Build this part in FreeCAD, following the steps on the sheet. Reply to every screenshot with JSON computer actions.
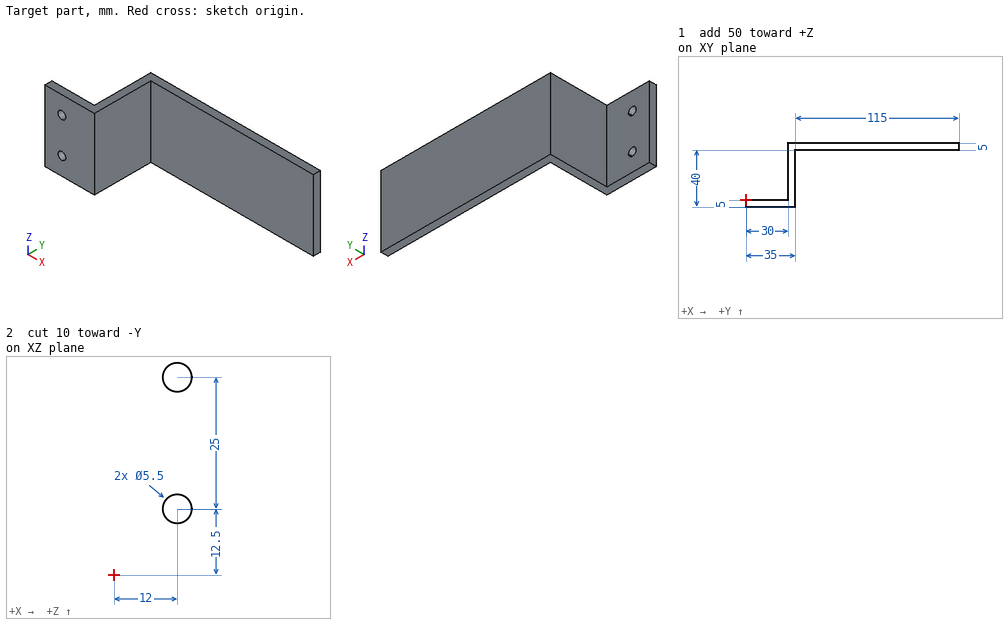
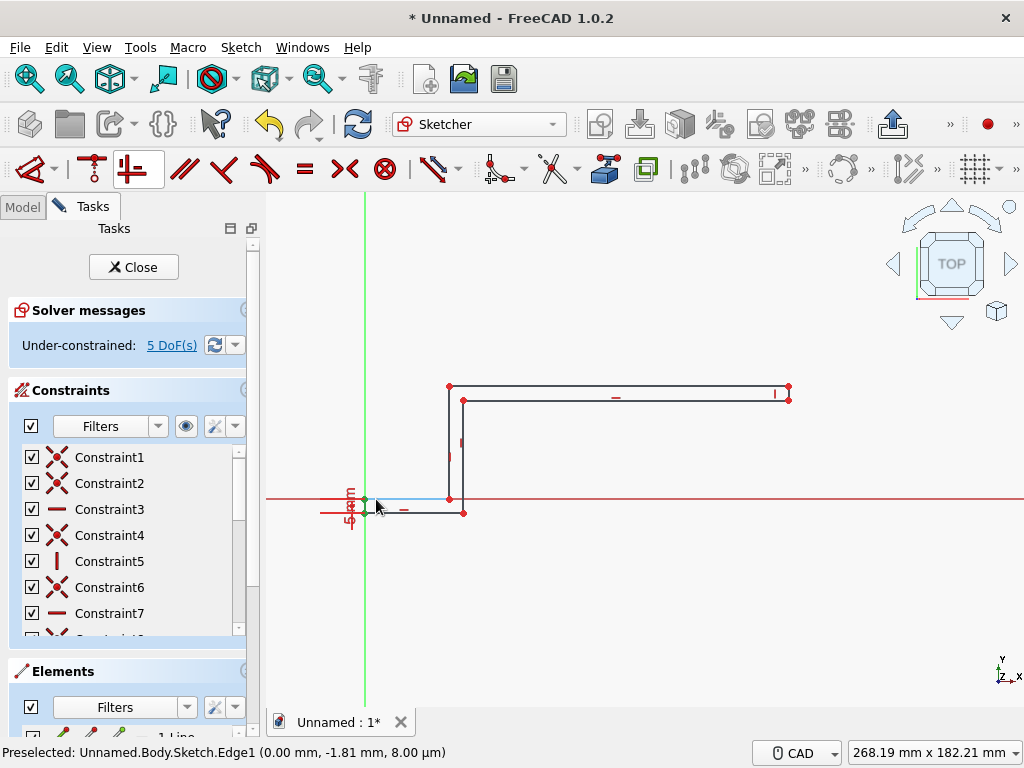
{"action": "scroll", "coordinate": [789, 396], "scroll_direction": "up", "scroll_amount": 6}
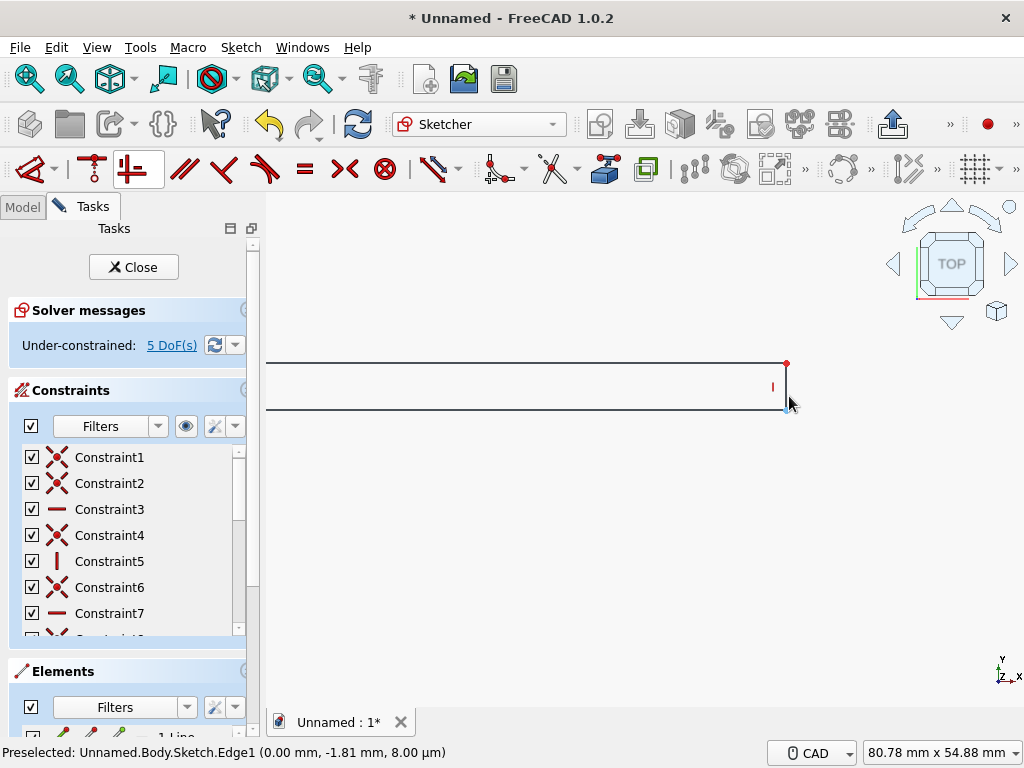
{"action": "left_click", "coordinate": [786, 396]}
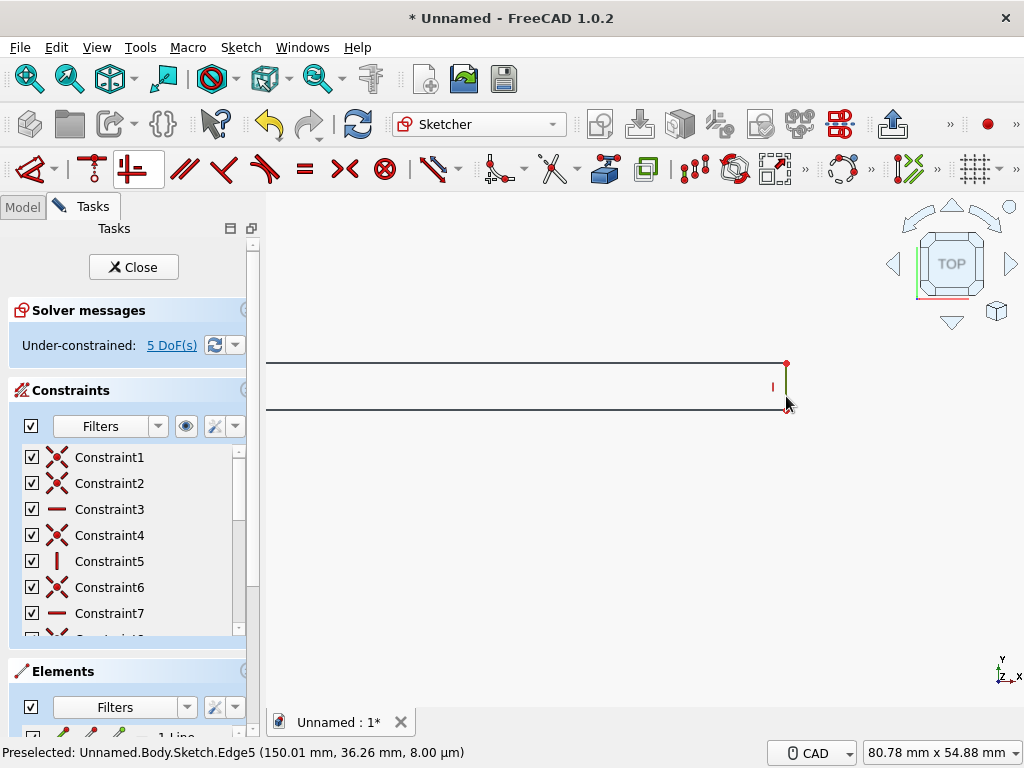
{"action": "key", "text": "i"}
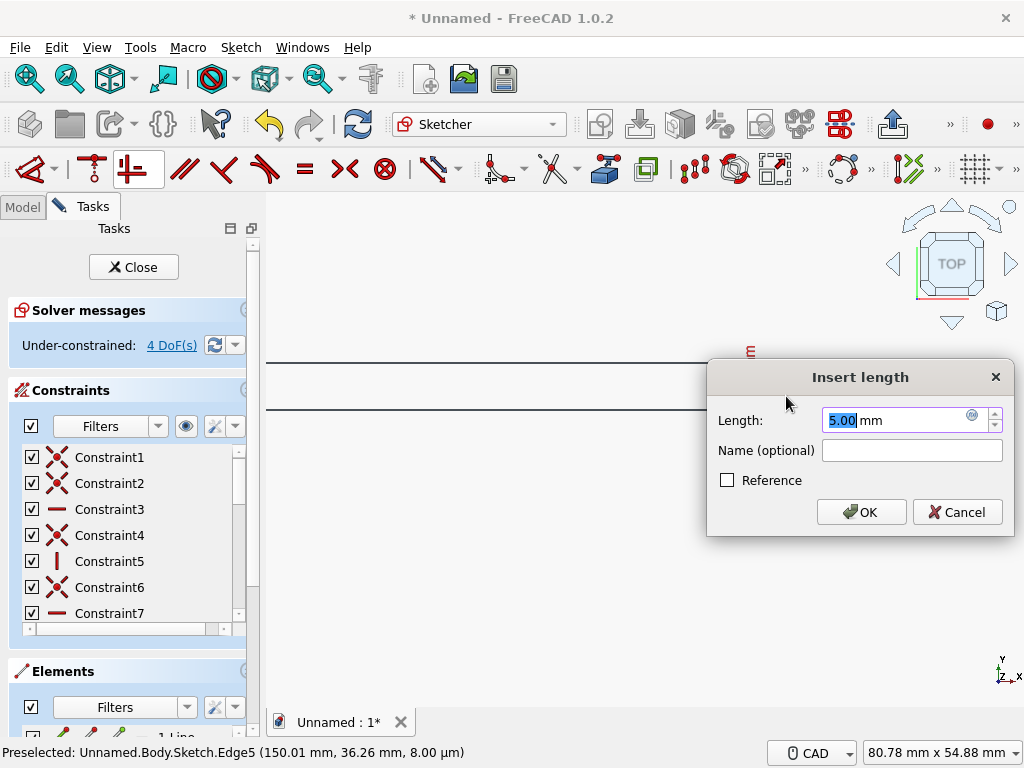
{"action": "type", "text": "5"}
{"action": "key", "text": "Return"}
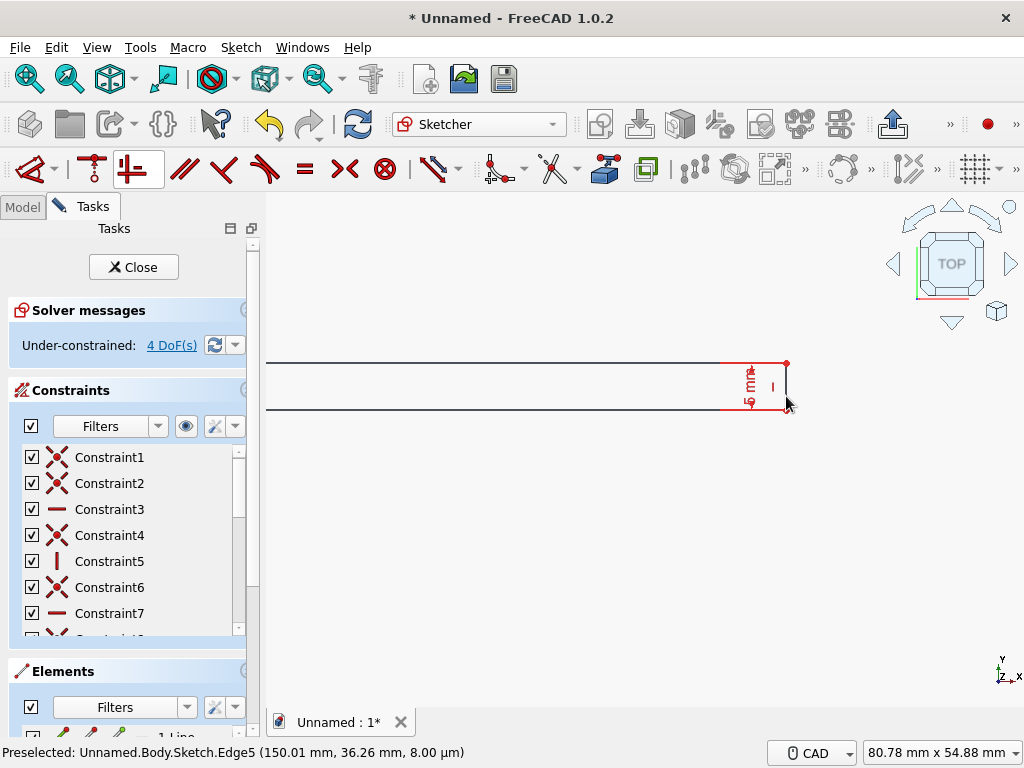
{"action": "scroll", "coordinate": [789, 396], "scroll_direction": "down", "scroll_amount": 6}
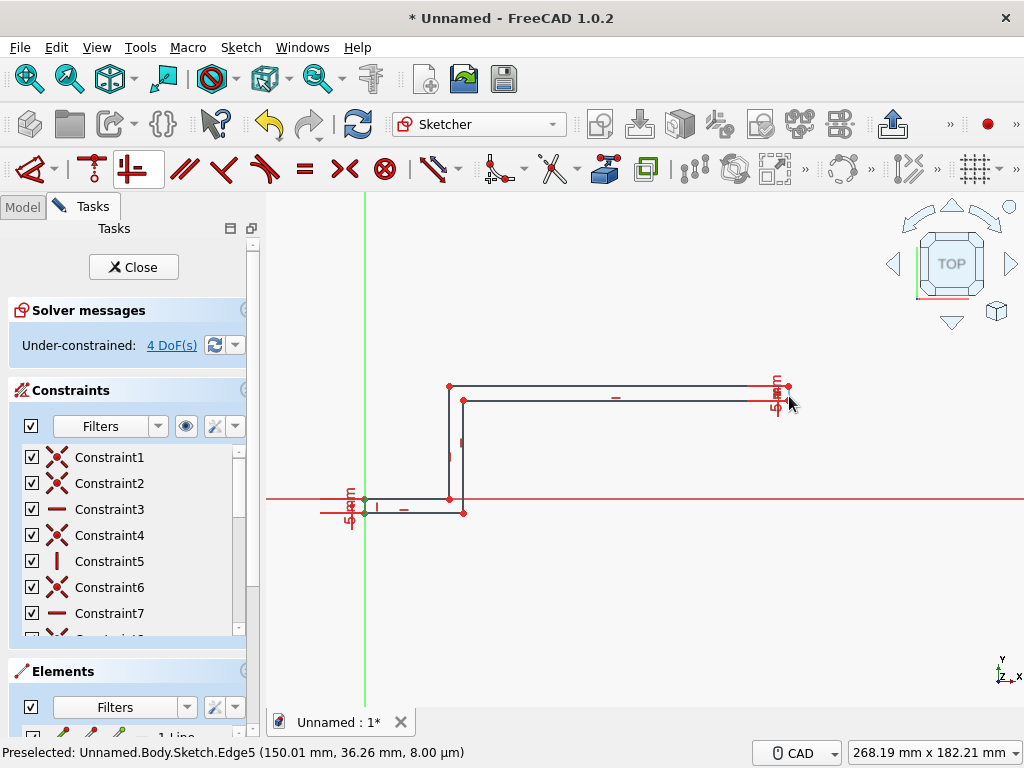
{"action": "left_click", "coordinate": [394, 513]}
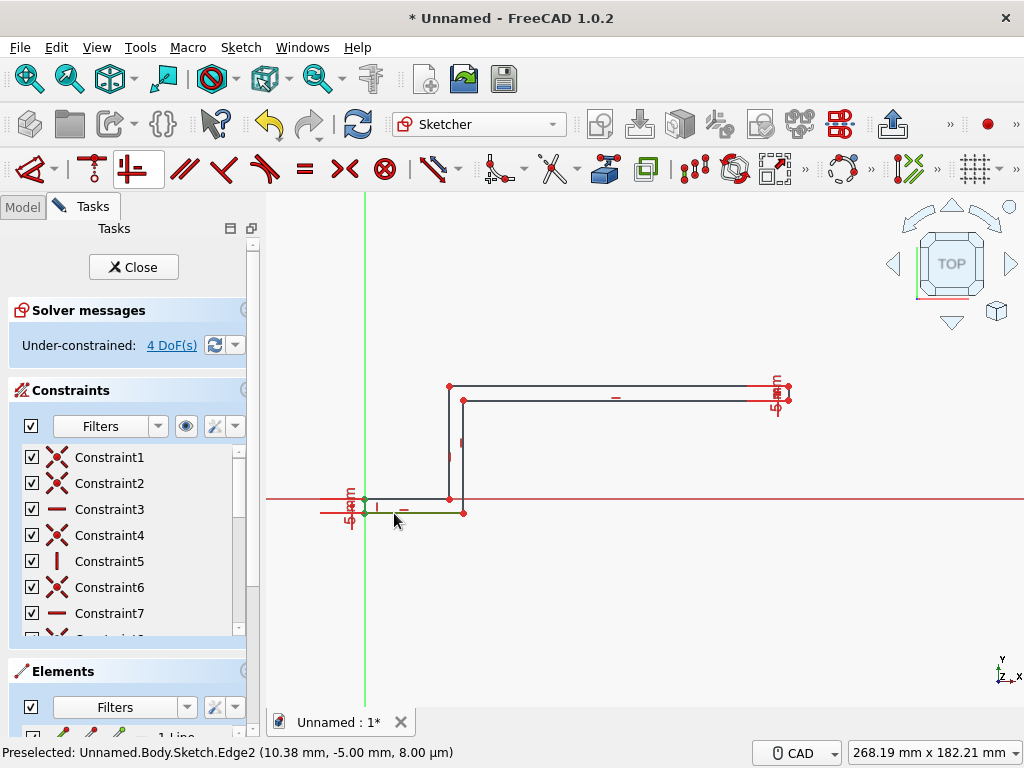
{"action": "key", "text": "l"}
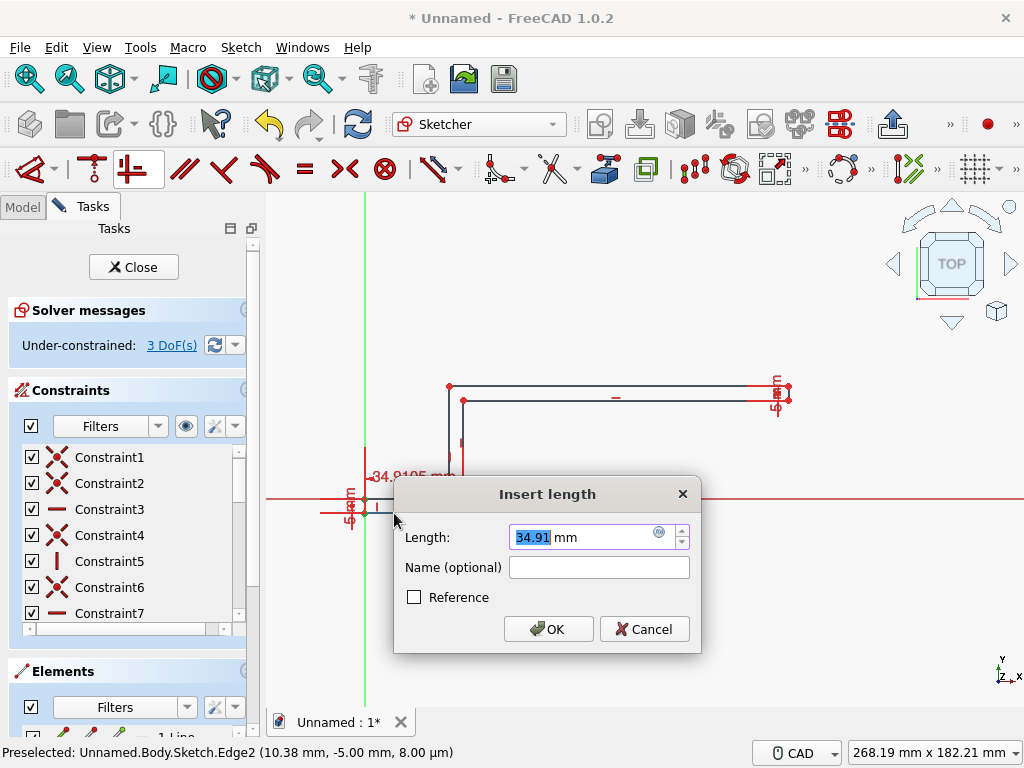
{"action": "type", "text": "35"}
{"action": "key", "text": "Return"}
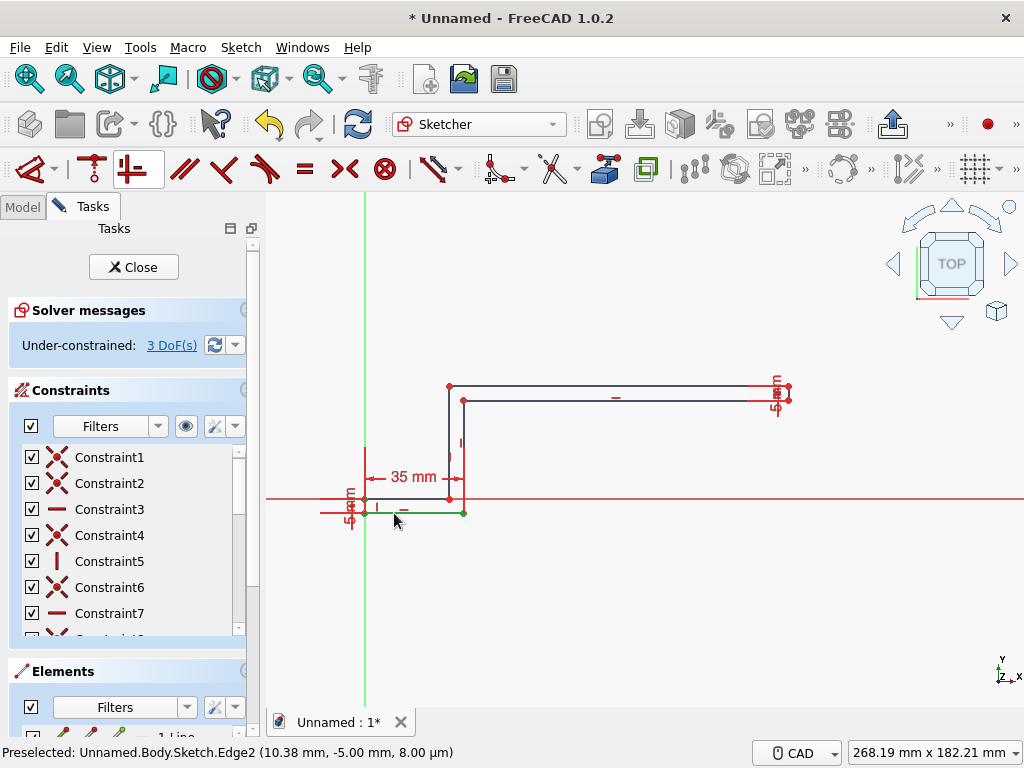
{"action": "left_click", "coordinate": [464, 479]}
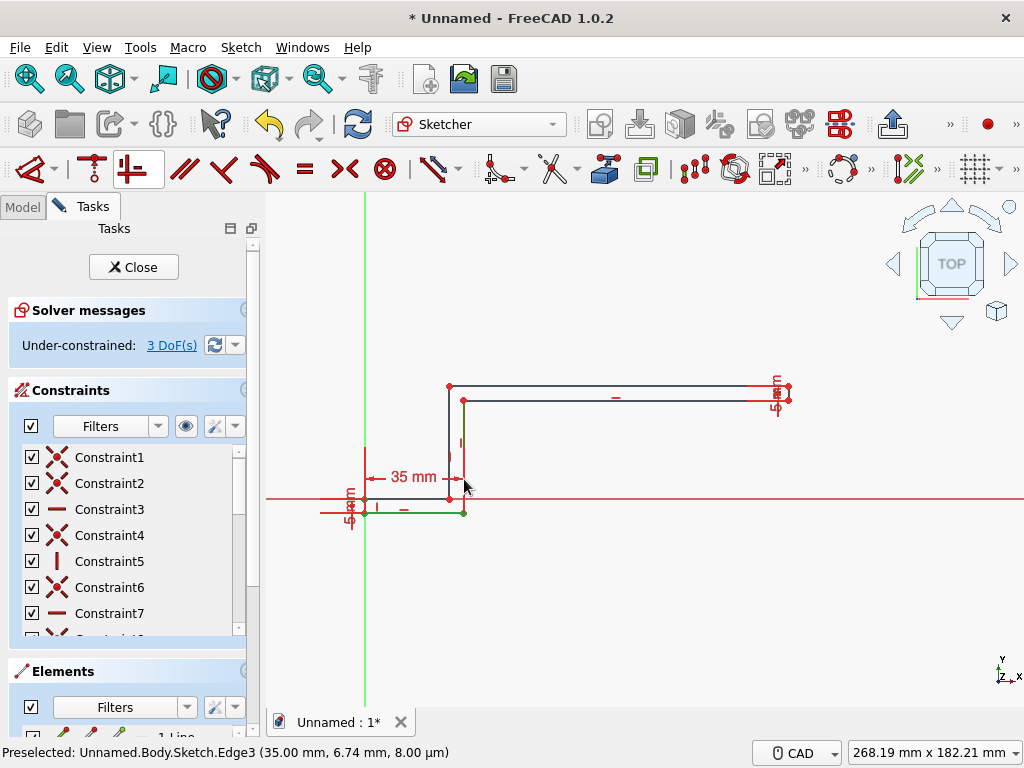
{"action": "left_click", "coordinate": [56, 170]}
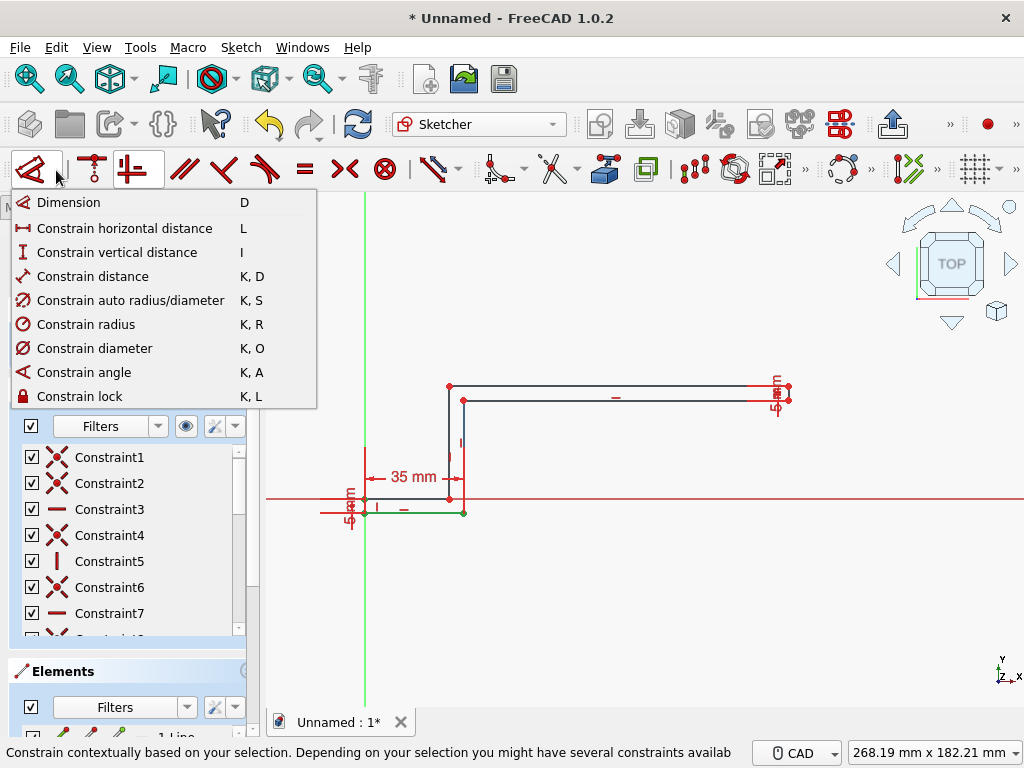
{"action": "left_click", "coordinate": [164, 252]}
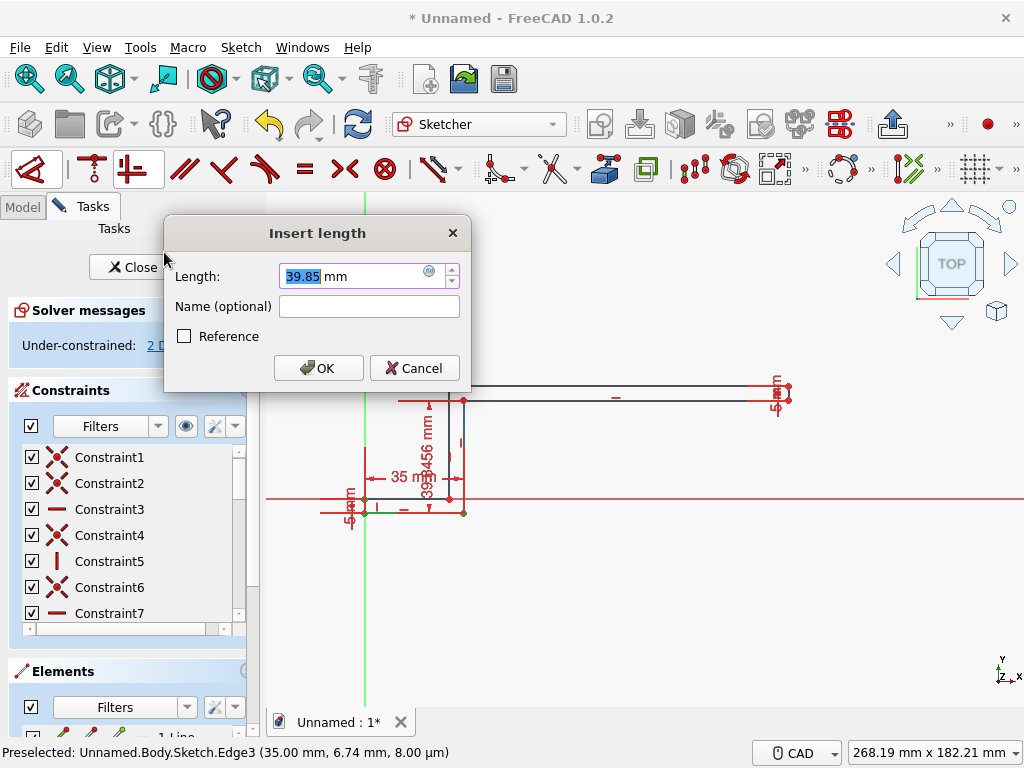
{"action": "type", "text": "40"}
{"action": "key", "text": "Return"}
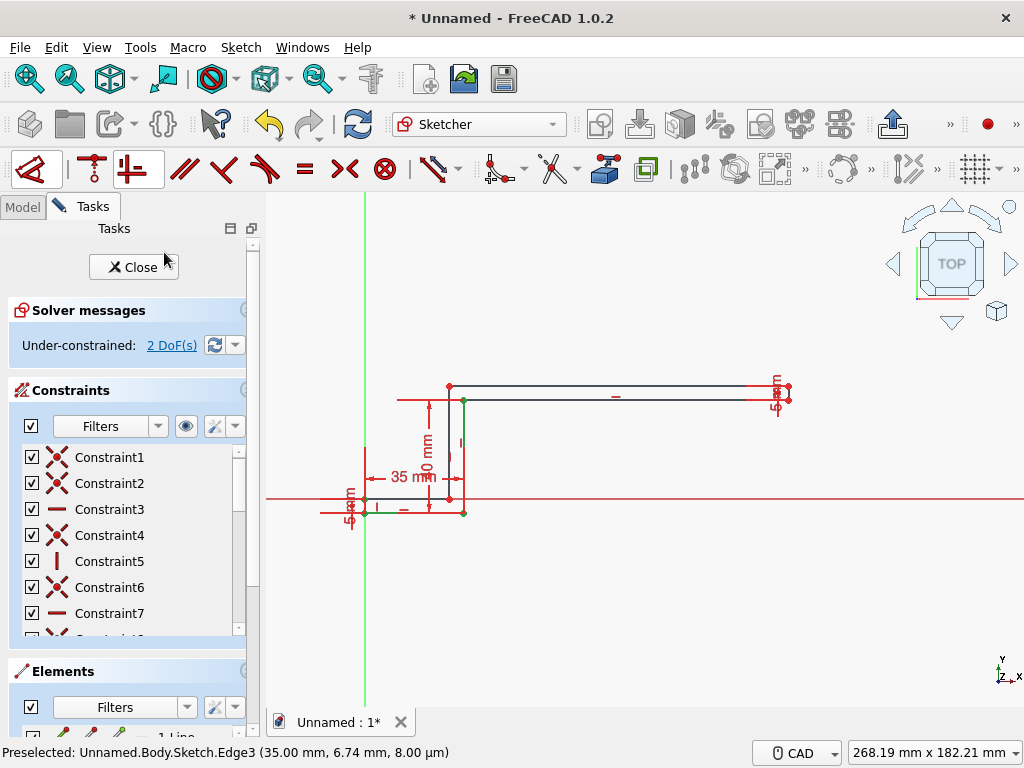
{"action": "left_click", "coordinate": [424, 499]}